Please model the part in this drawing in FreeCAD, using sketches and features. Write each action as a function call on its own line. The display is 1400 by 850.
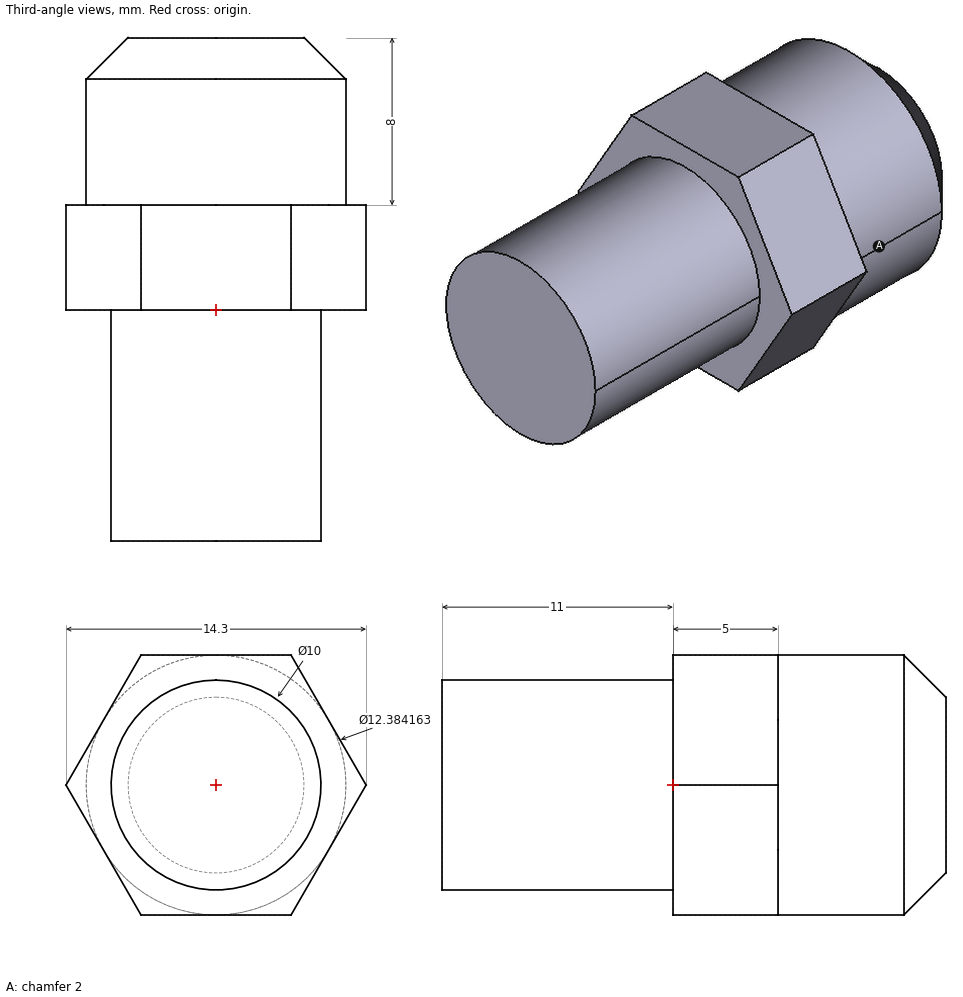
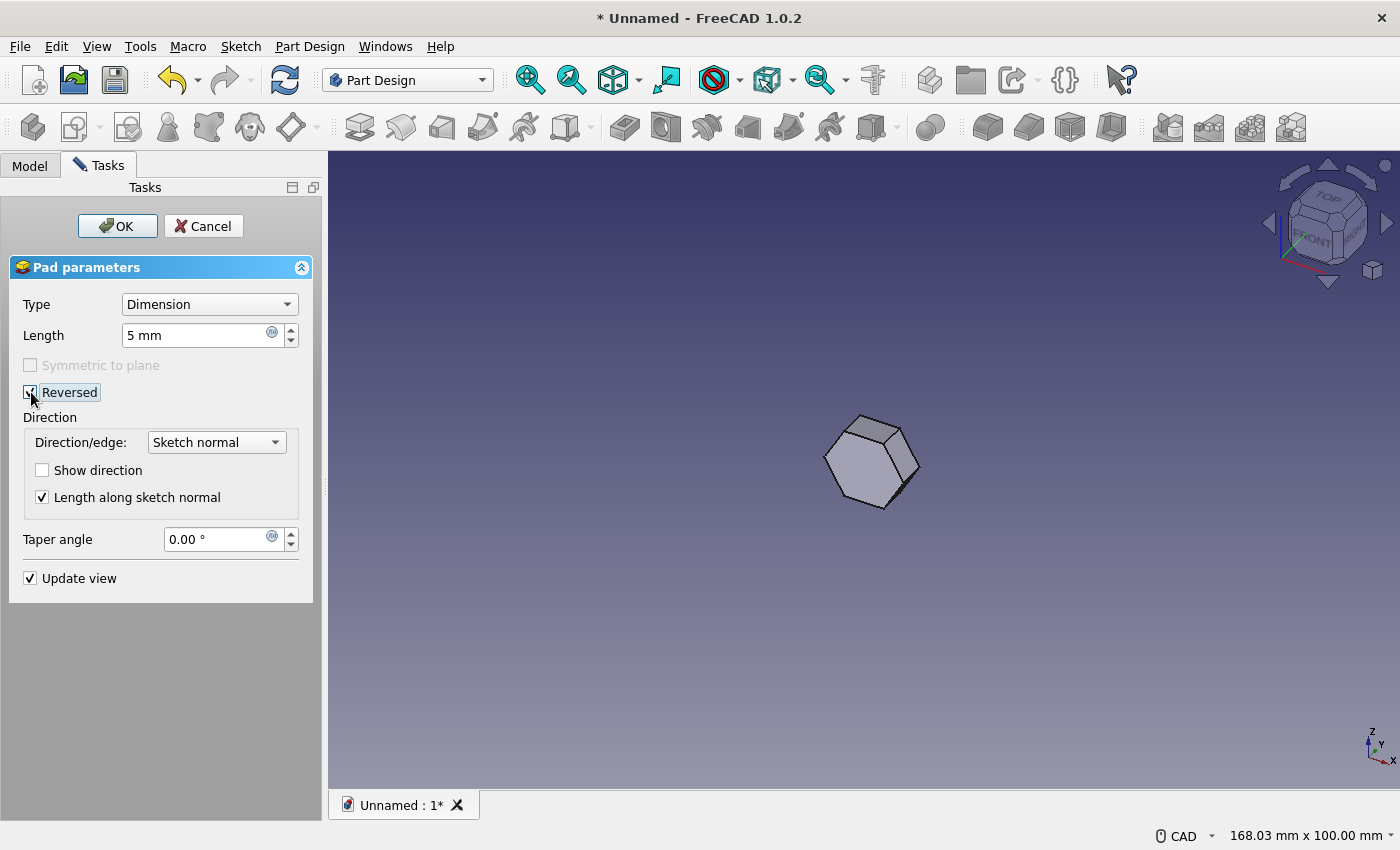
click(118, 226)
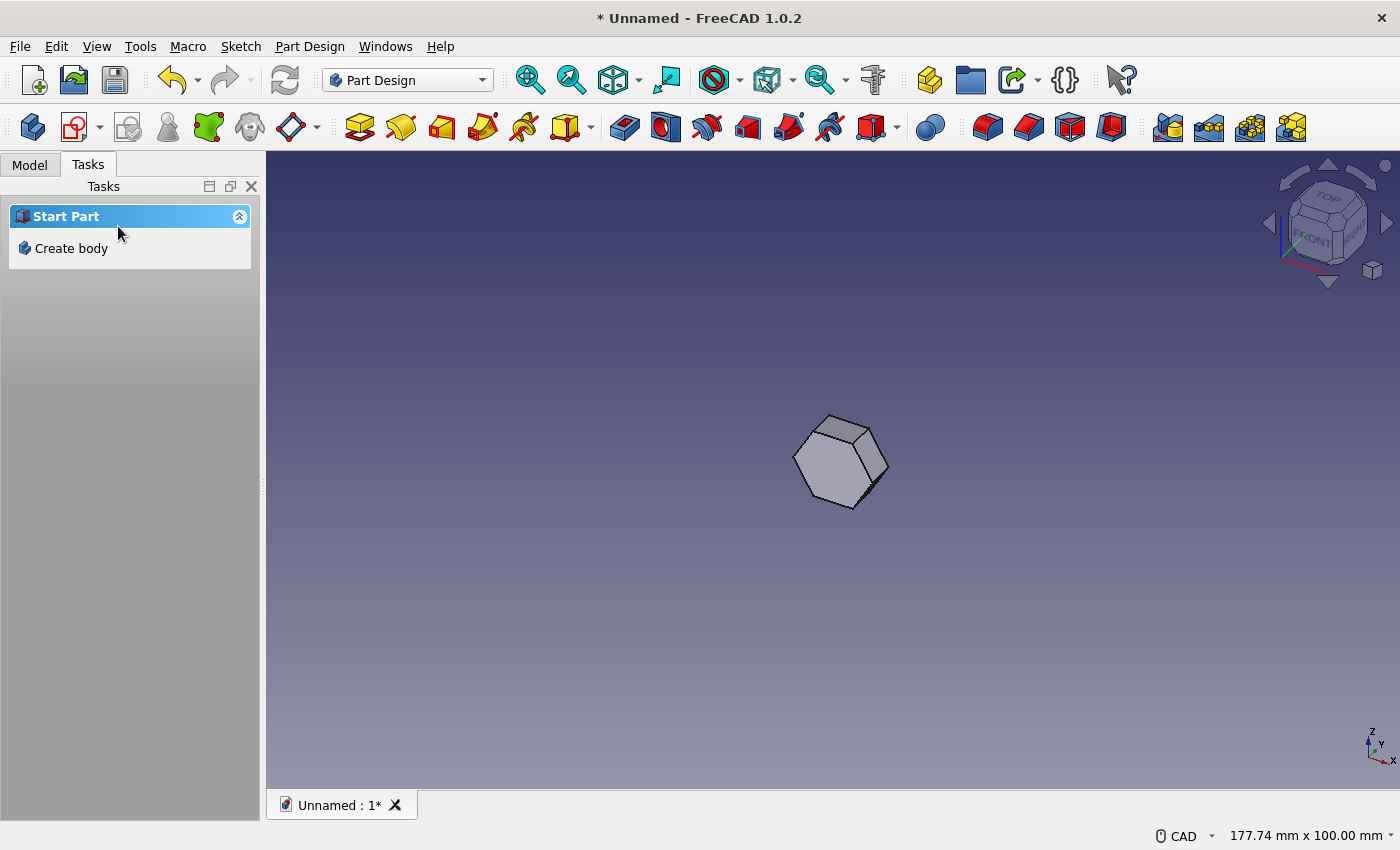
click(531, 80)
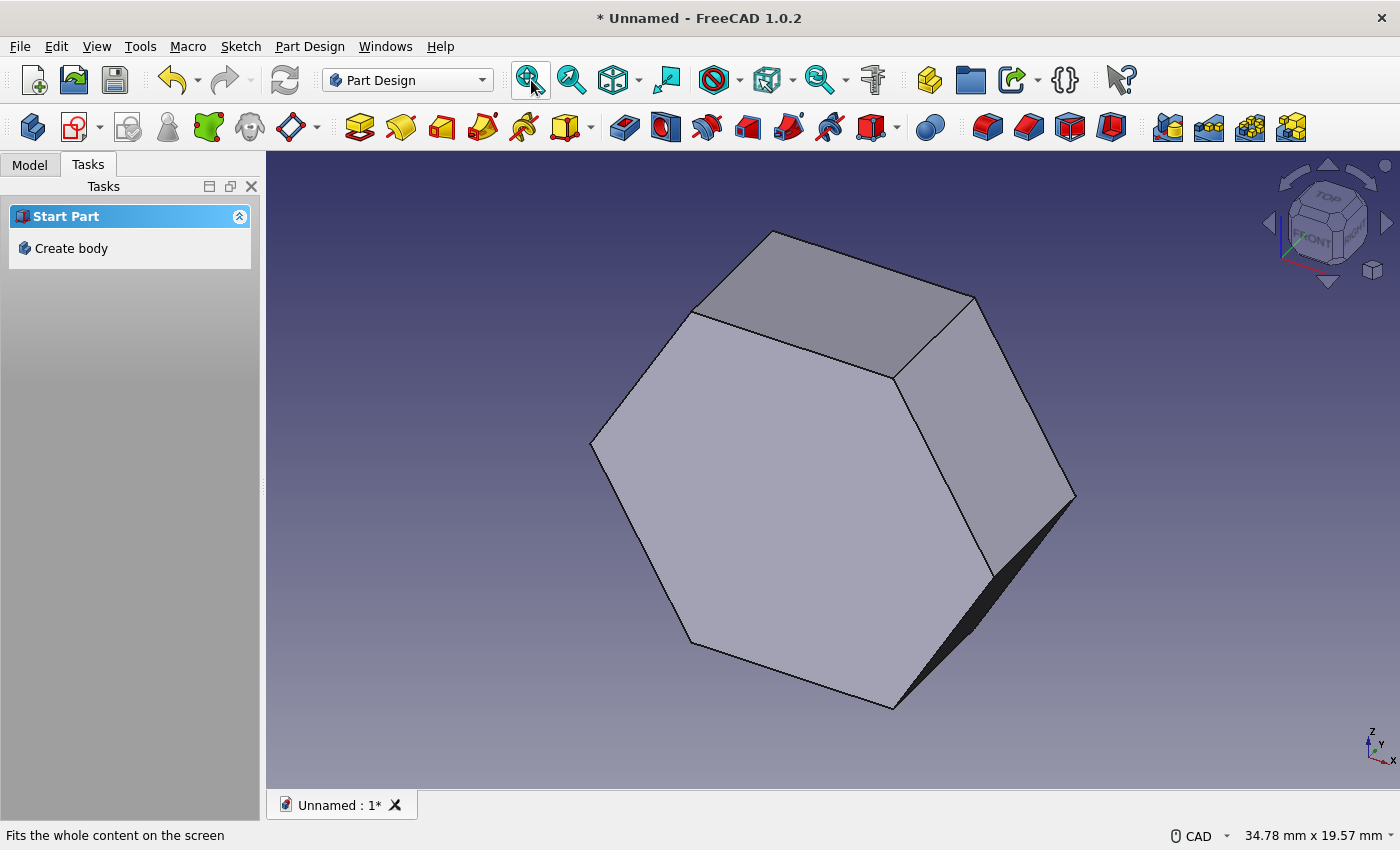
key(4)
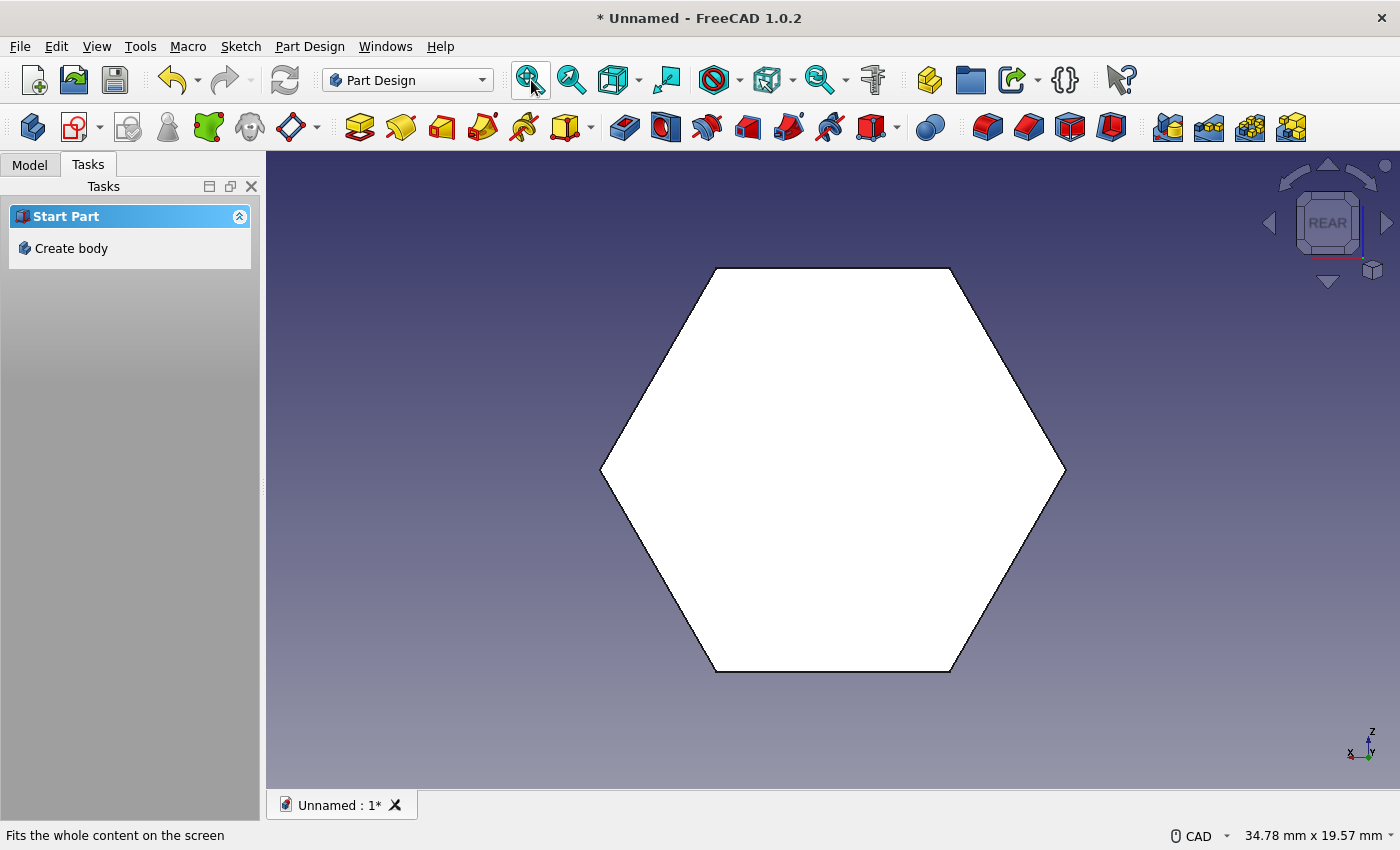
click(833, 469)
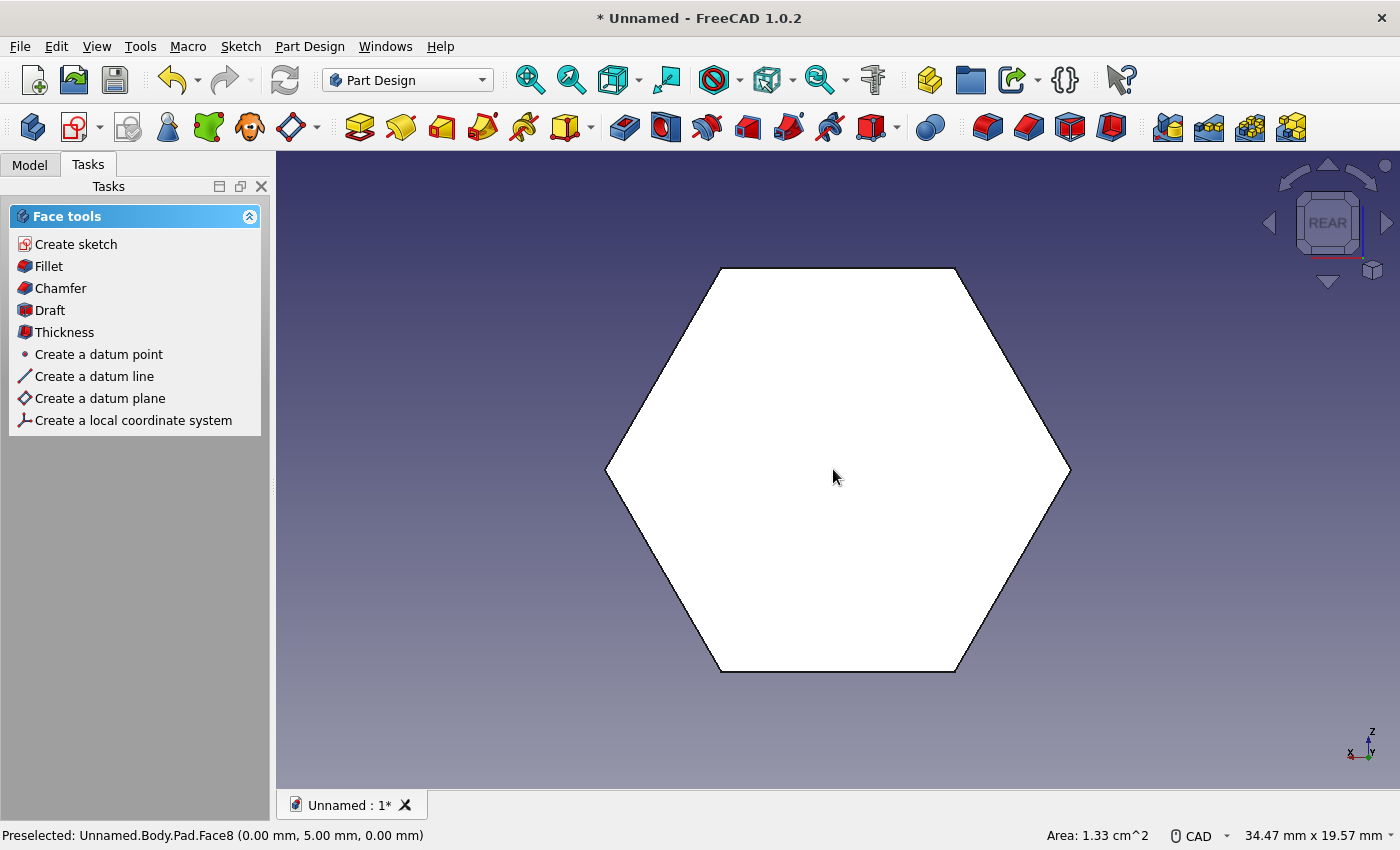
click(74, 128)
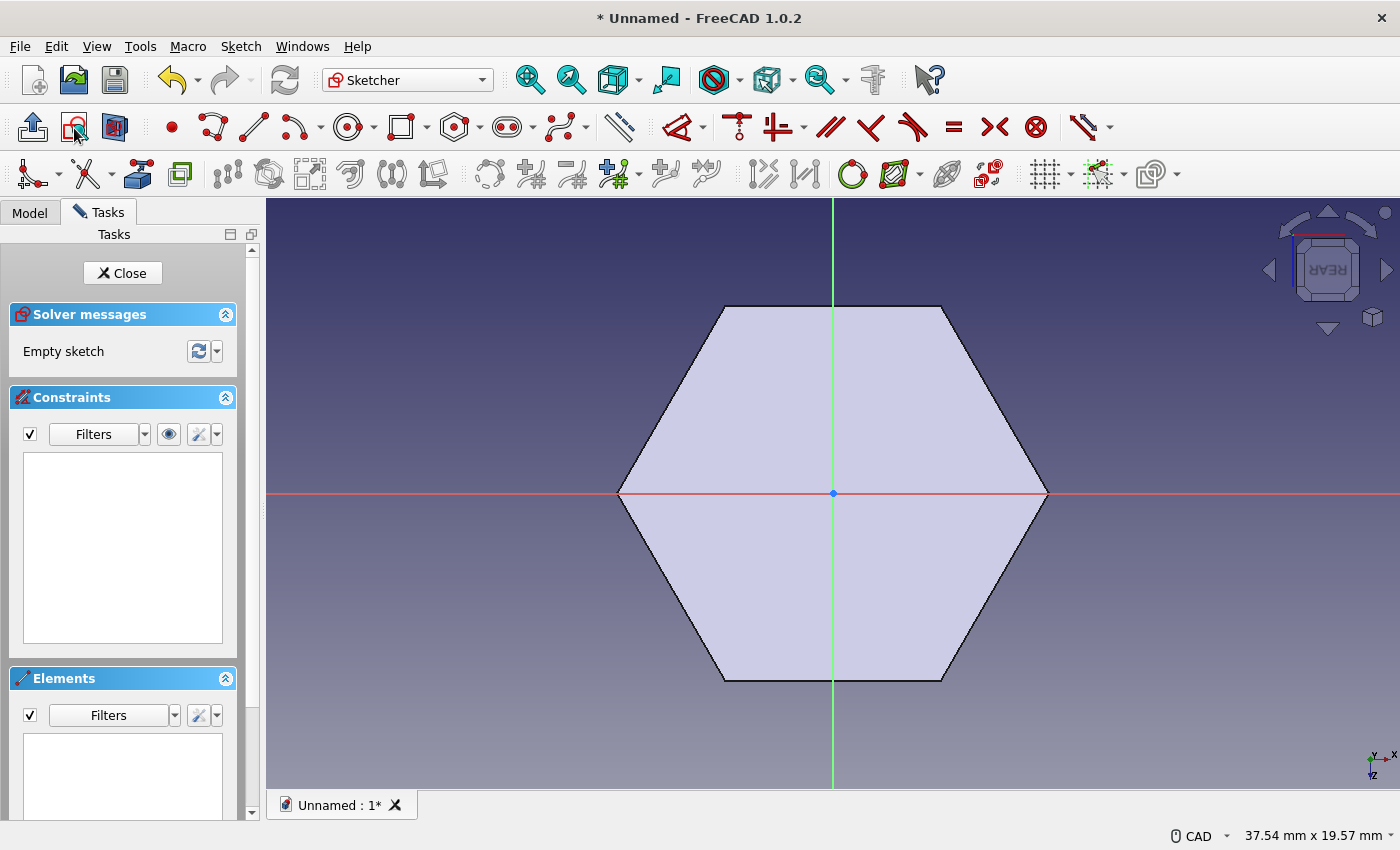
click(348, 128)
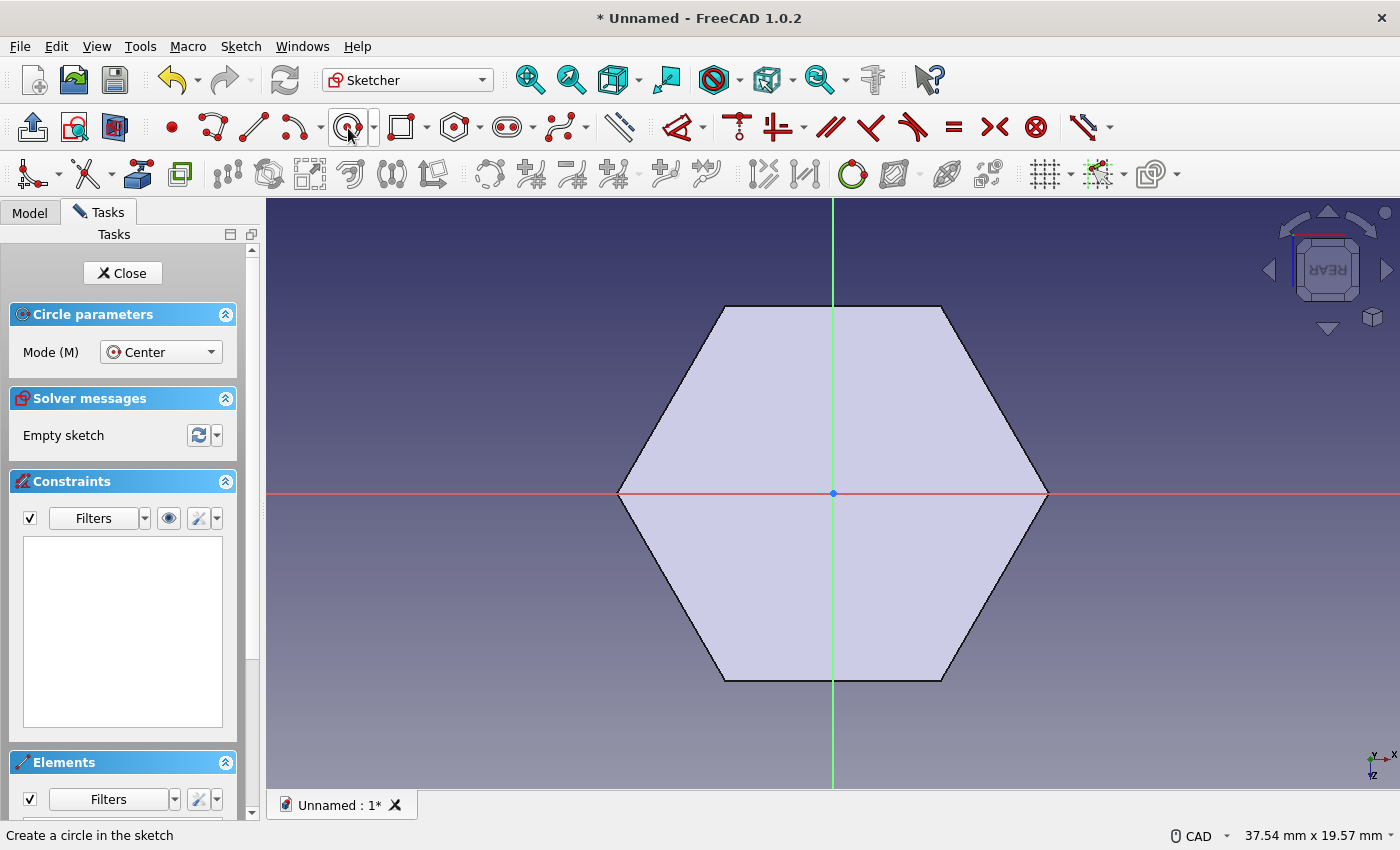
click(833, 494)
click(965, 361)
key(Escape)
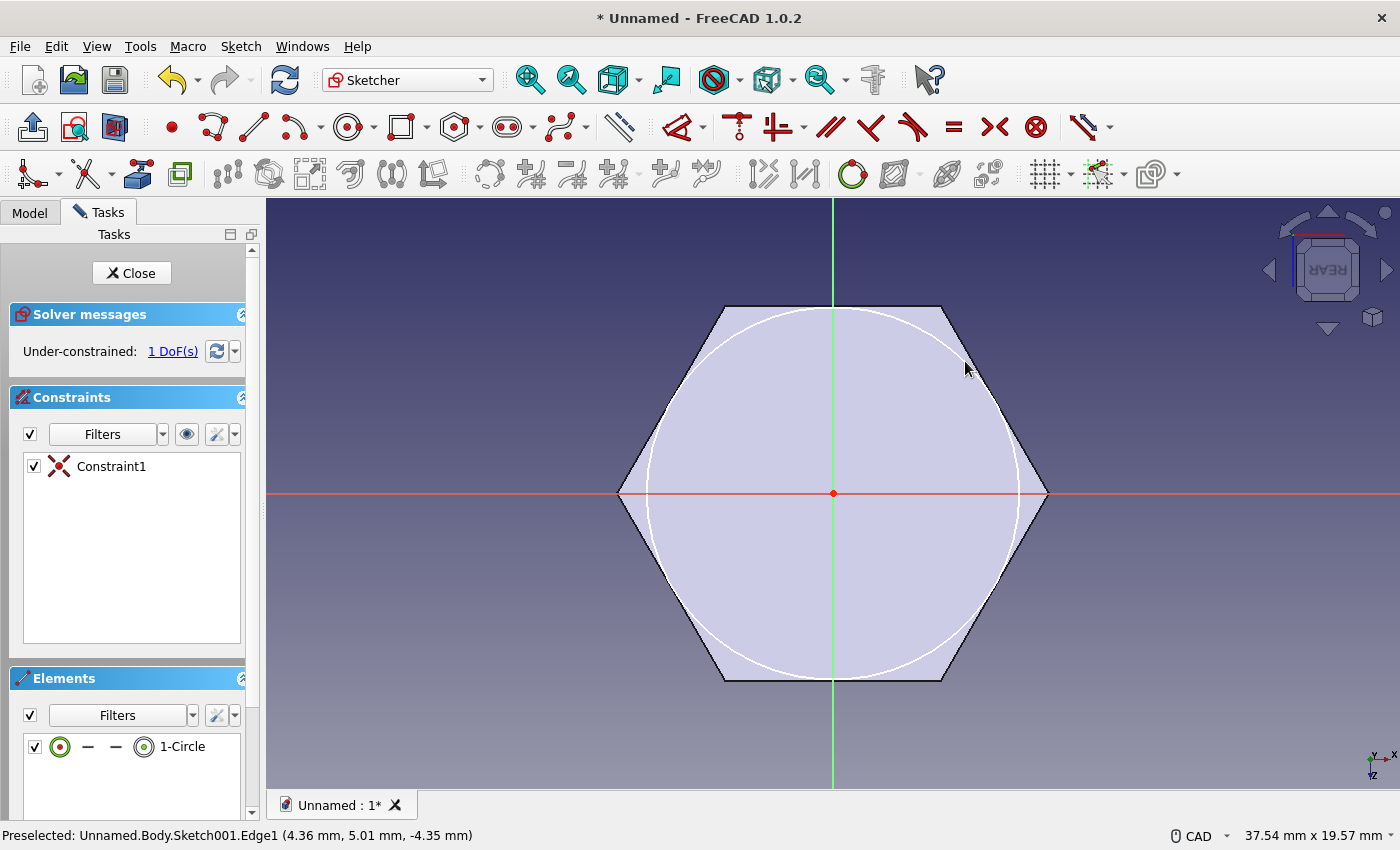
click(676, 128)